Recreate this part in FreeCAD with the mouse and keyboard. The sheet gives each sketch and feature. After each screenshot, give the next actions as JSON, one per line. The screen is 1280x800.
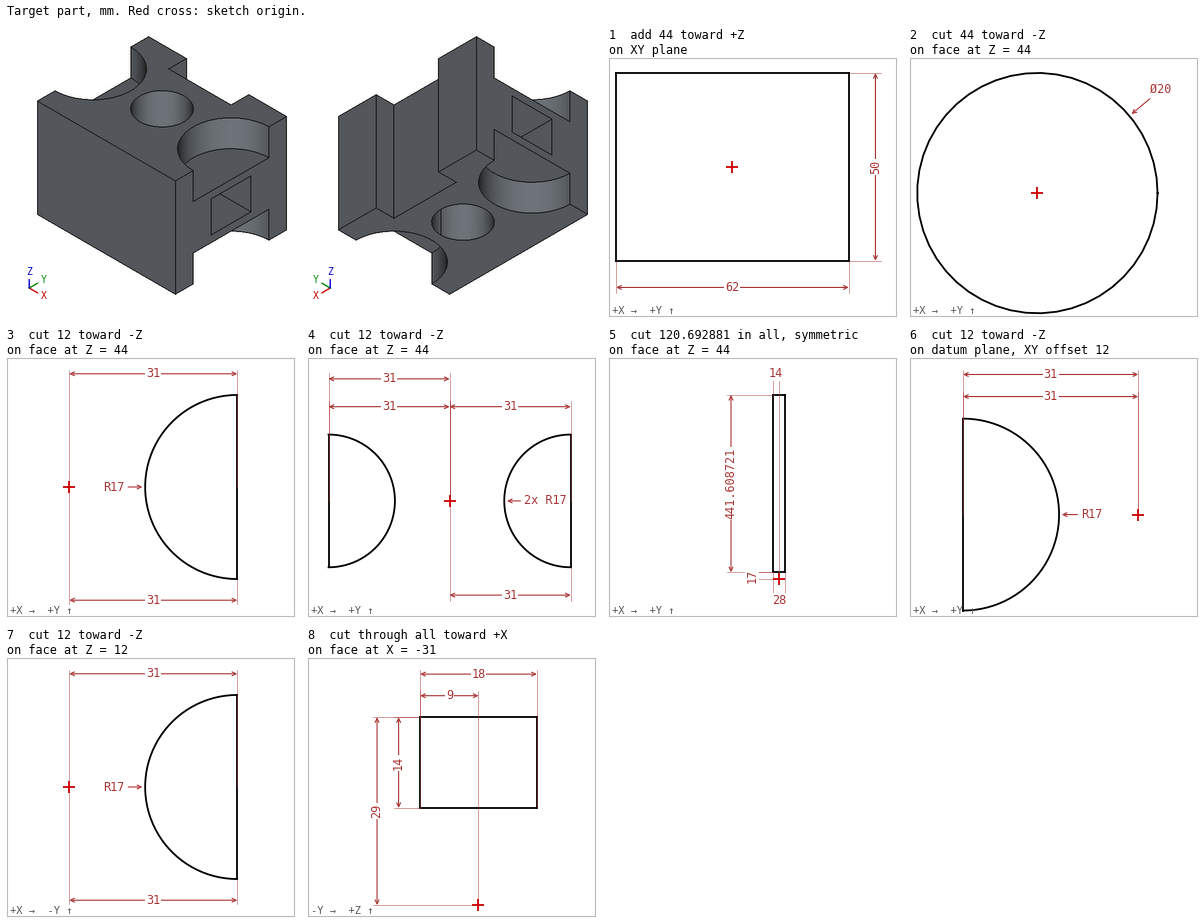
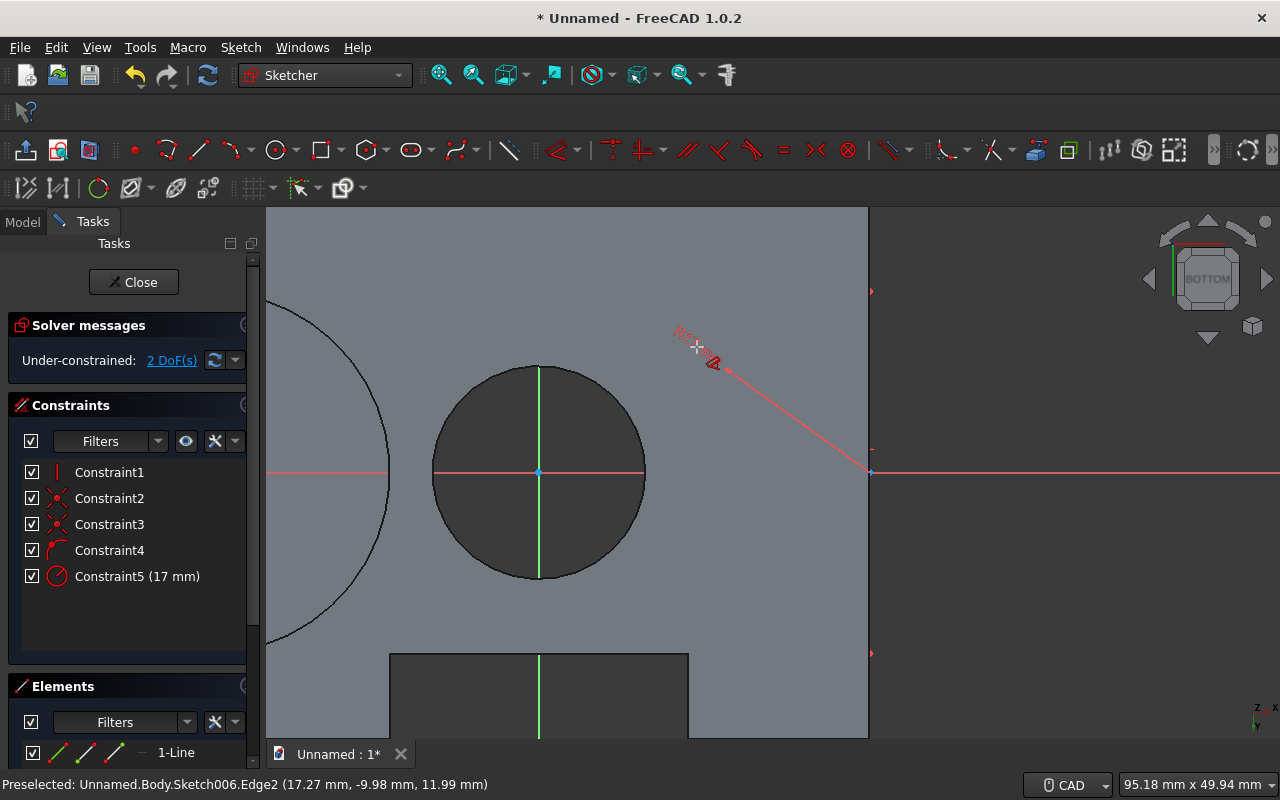
{"action": "left_click", "coordinate": [869, 654]}
{"action": "left_click", "coordinate": [704, 688]}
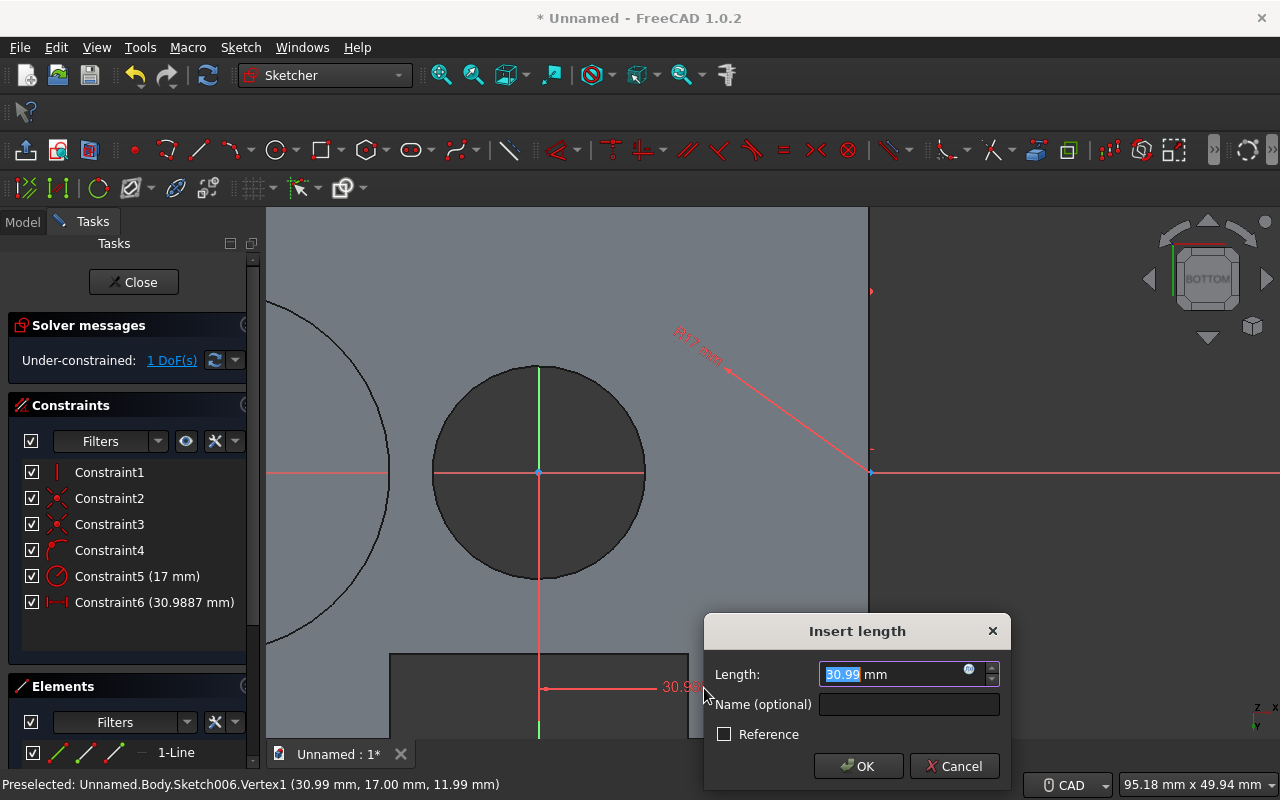
{"action": "type", "text": "31"}
{"action": "key", "text": "Return"}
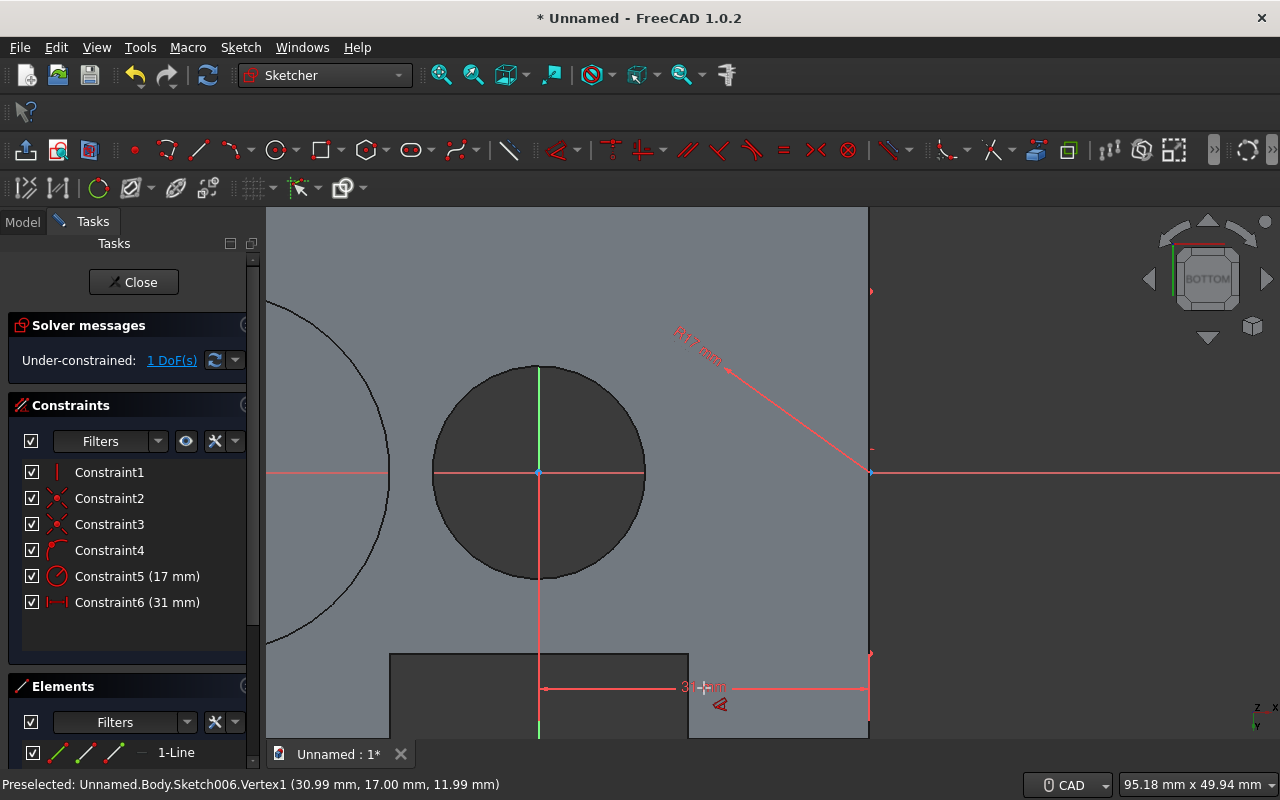
{"action": "left_click", "coordinate": [870, 473]}
{"action": "left_click", "coordinate": [628, 507]}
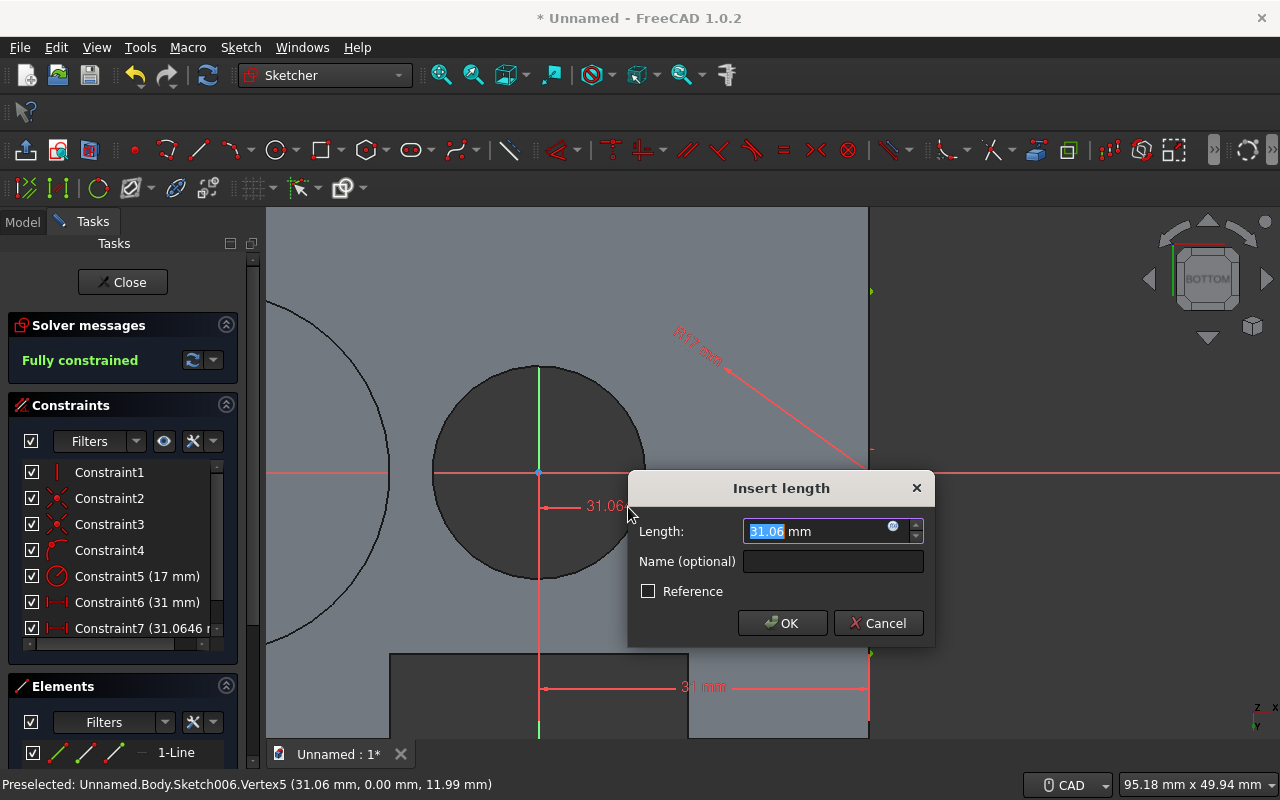
{"action": "type", "text": "31"}
{"action": "key", "text": "Return"}
{"action": "key", "text": "Escape"}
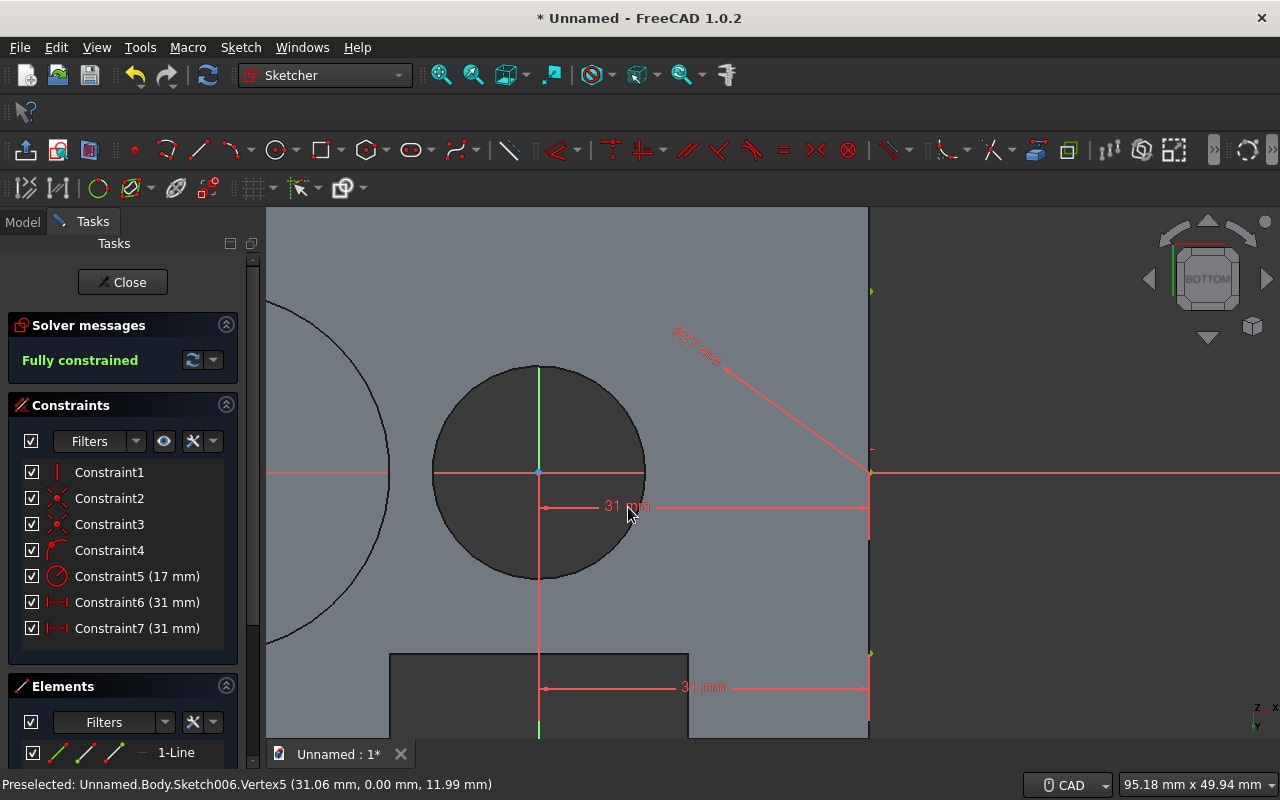
{"action": "left_click", "coordinate": [123, 282]}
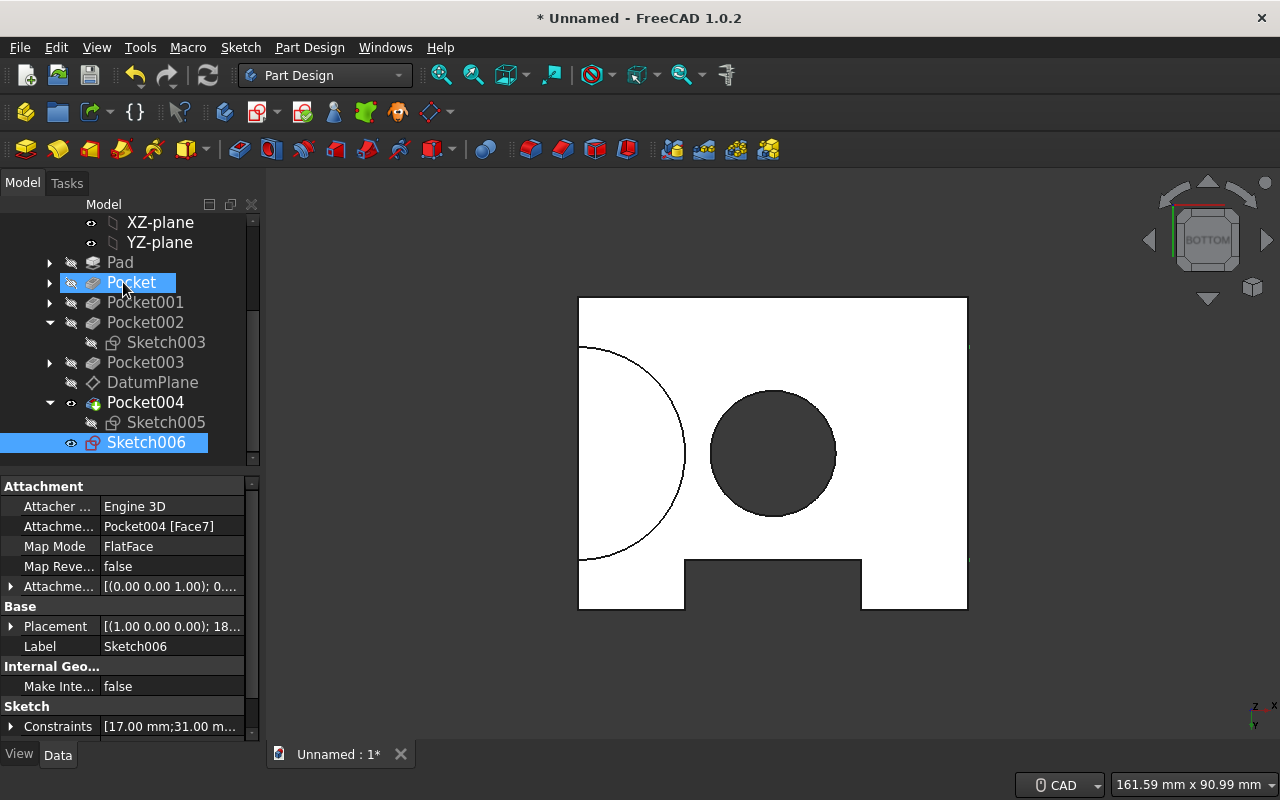
{"action": "left_click", "coordinate": [240, 150]}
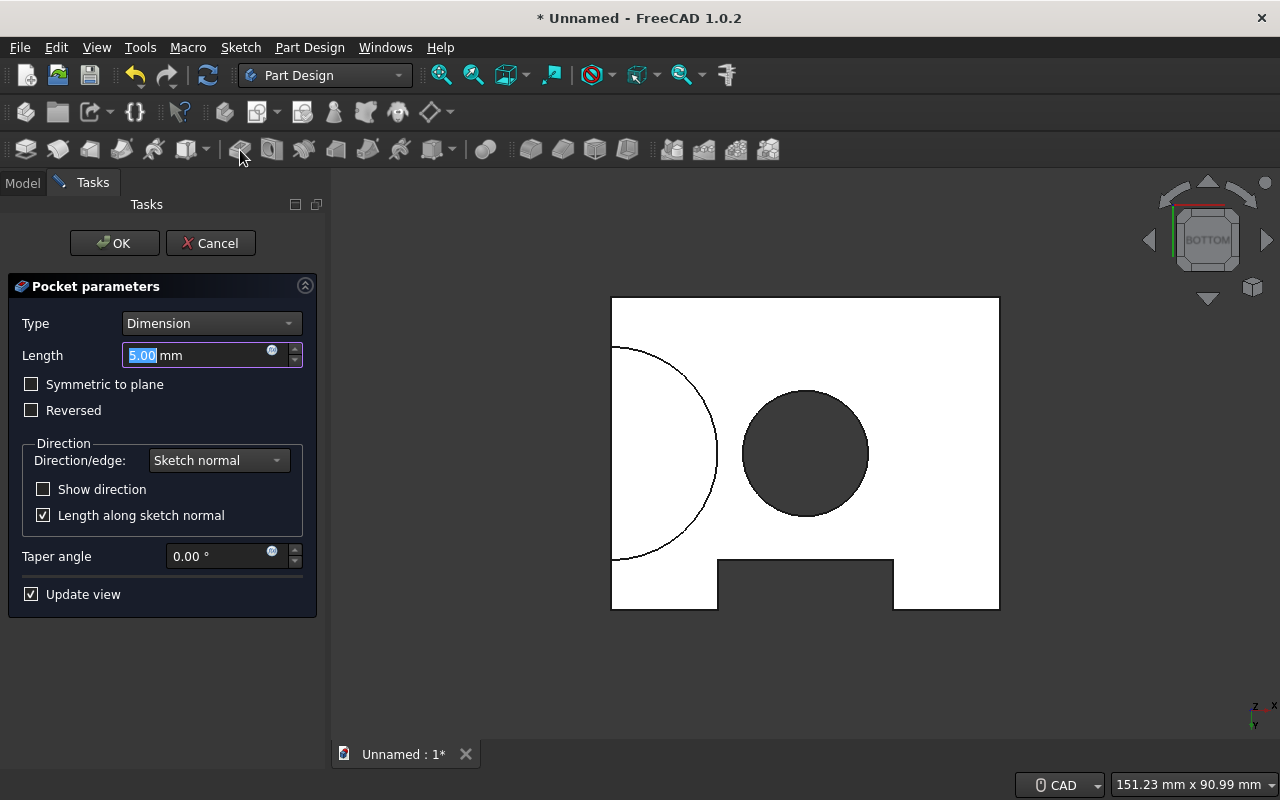
{"action": "type", "text": "12"}
{"action": "key", "text": "Tab"}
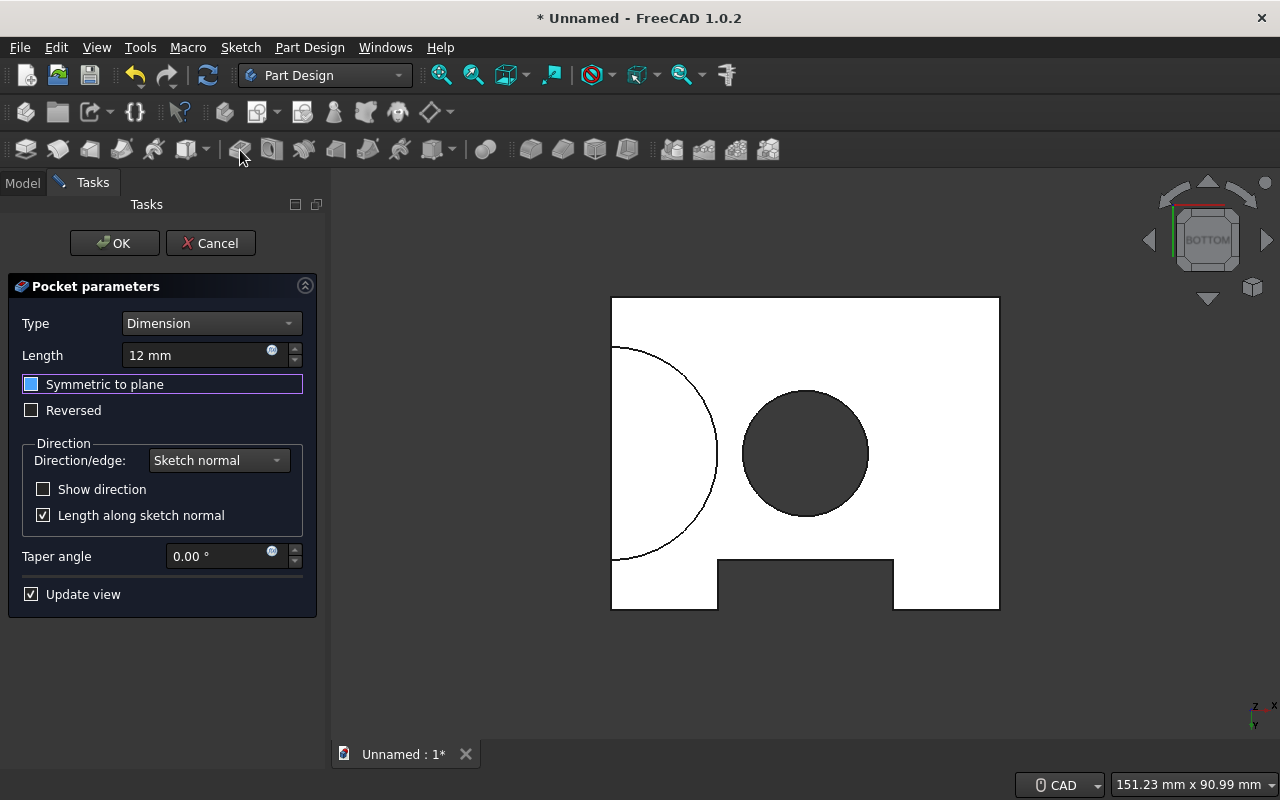
{"action": "left_click", "coordinate": [30, 410]}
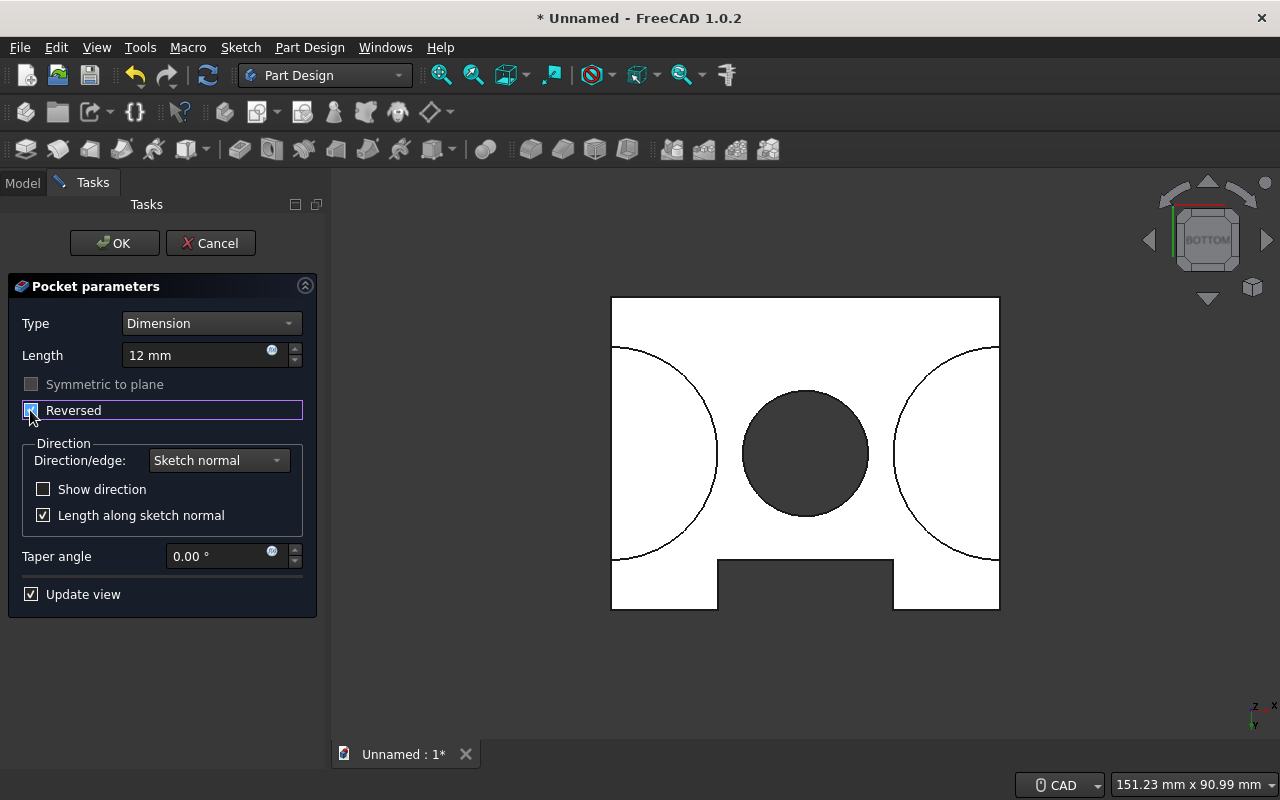
{"action": "left_click", "coordinate": [115, 243]}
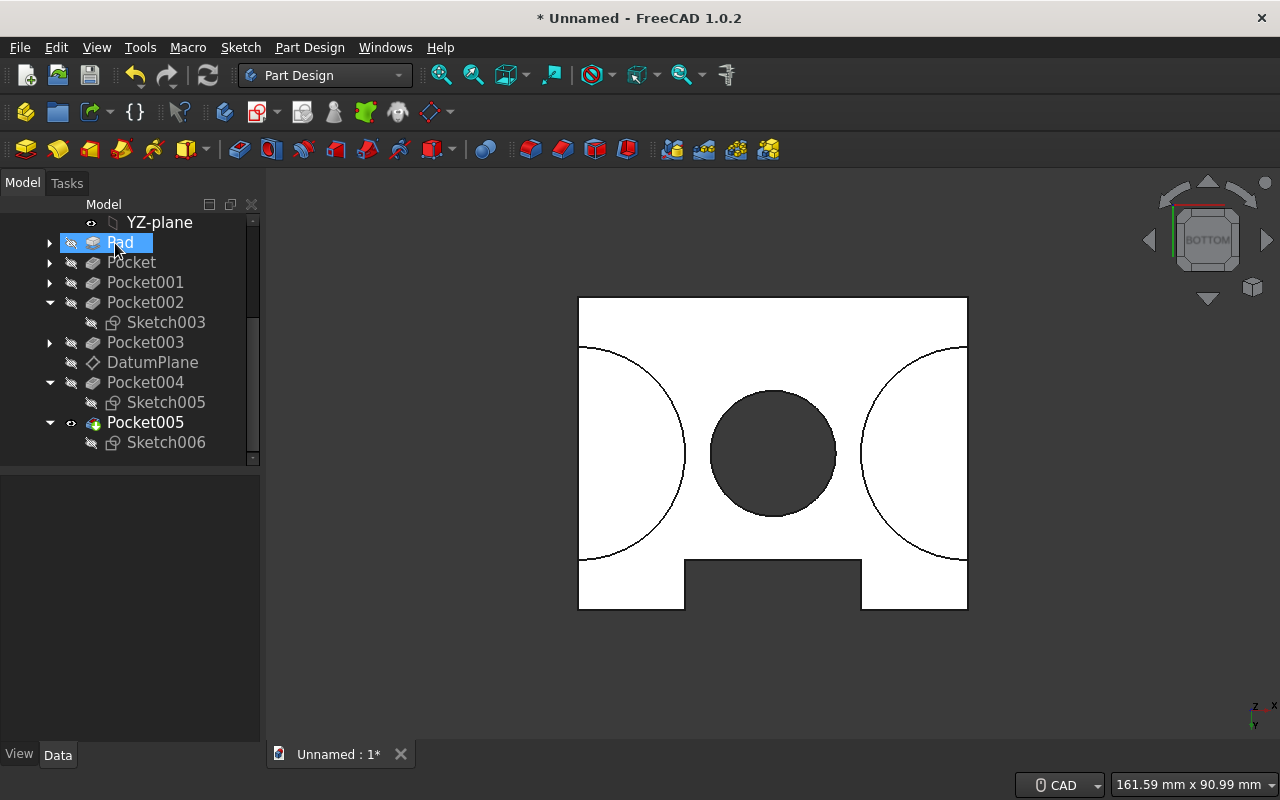
{"action": "key", "text": "6"}